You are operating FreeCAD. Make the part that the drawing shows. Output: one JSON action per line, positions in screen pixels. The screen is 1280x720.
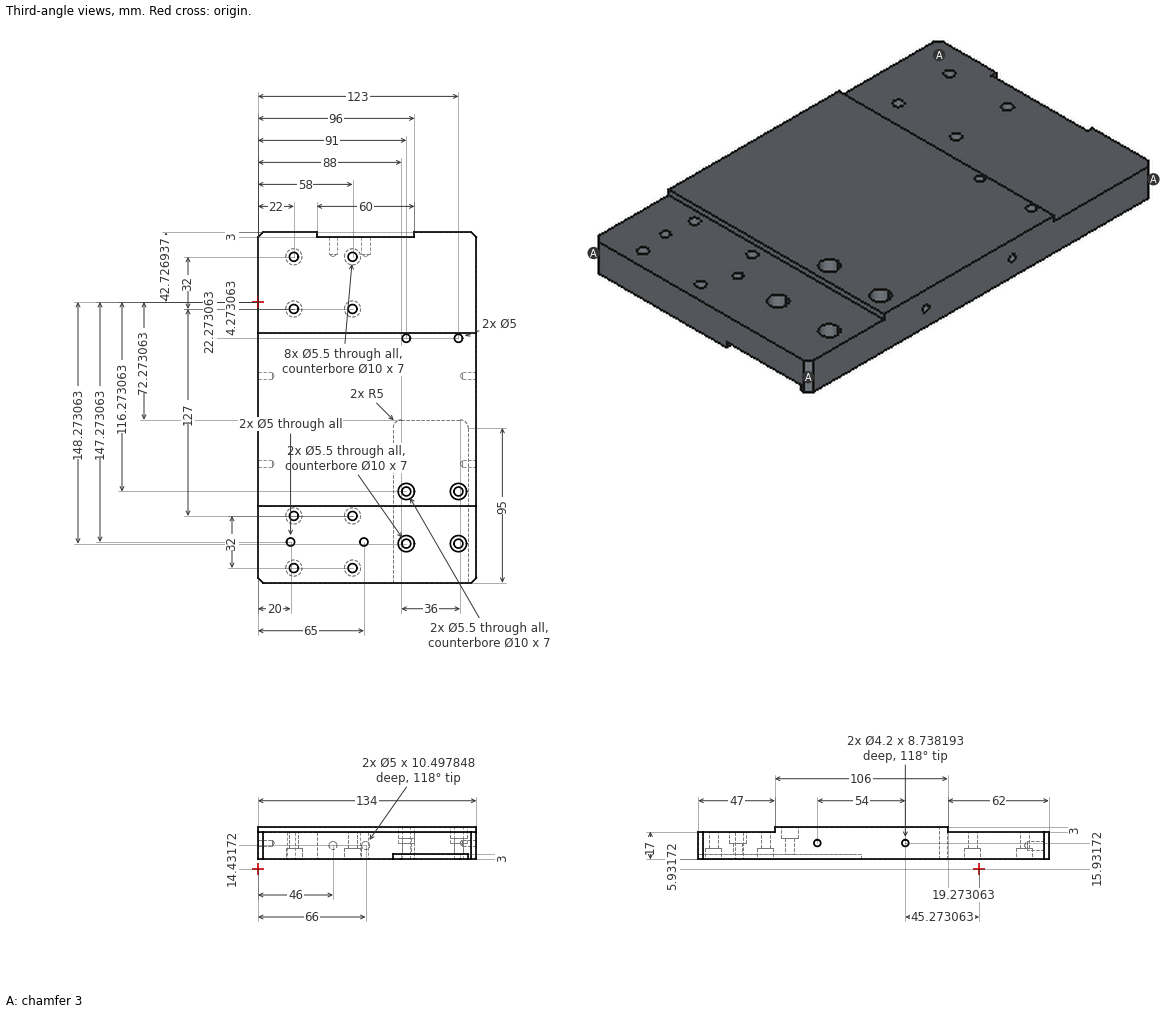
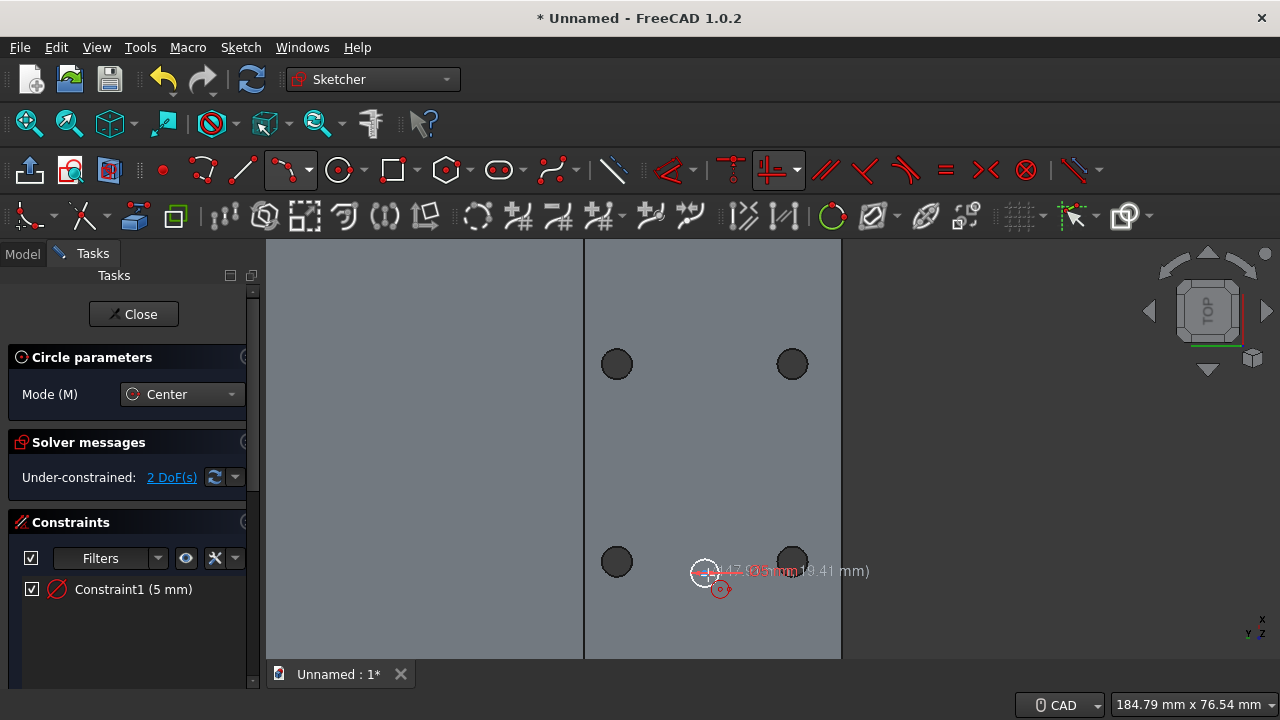
{"action": "scroll", "coordinate": [705, 326], "scroll_direction": "up", "scroll_amount": 3}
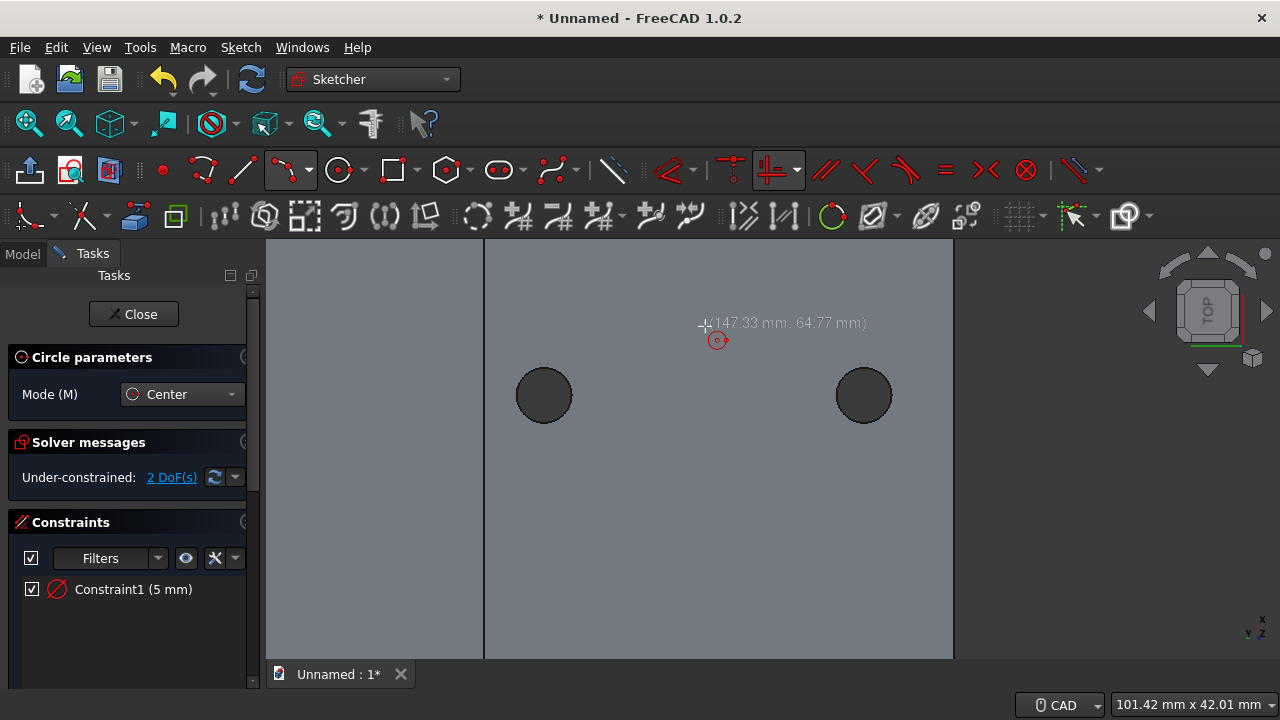
{"action": "left_click", "coordinate": [704, 325]}
{"action": "mouse_move", "coordinate": [722, 308]}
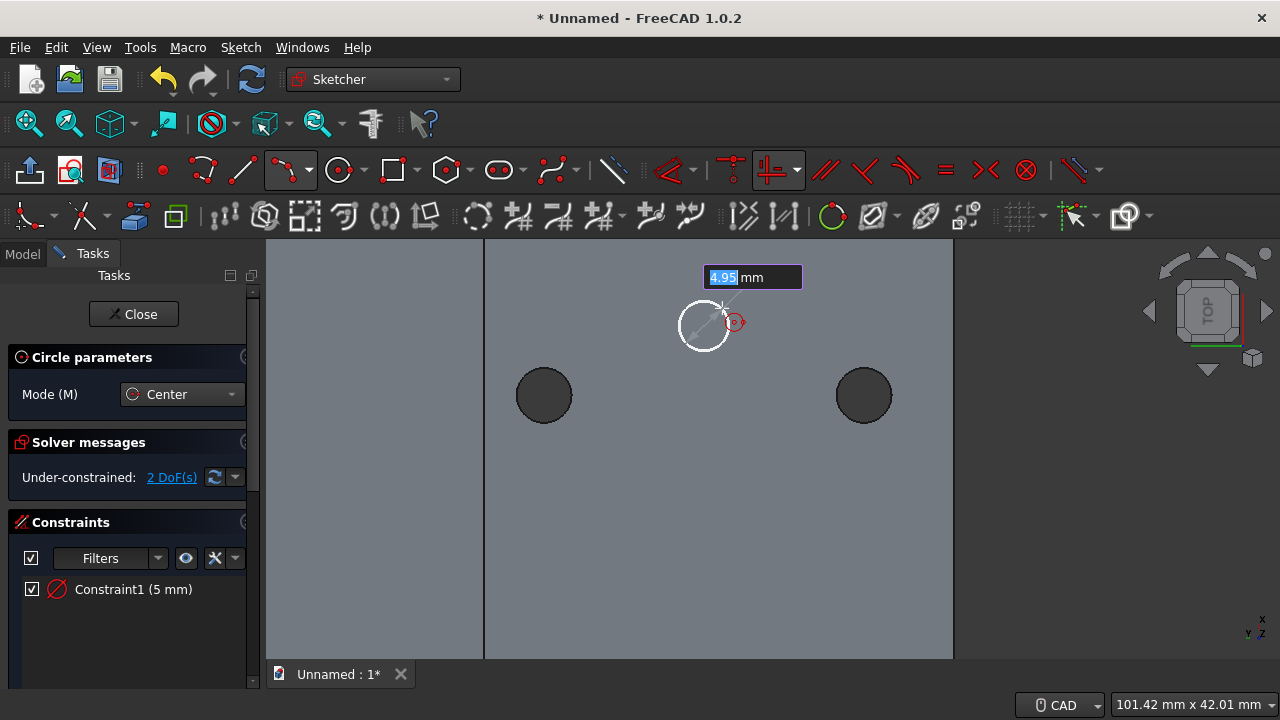
{"action": "type", "text": "5"}
{"action": "key", "text": "Return"}
{"action": "key", "text": "Escape"}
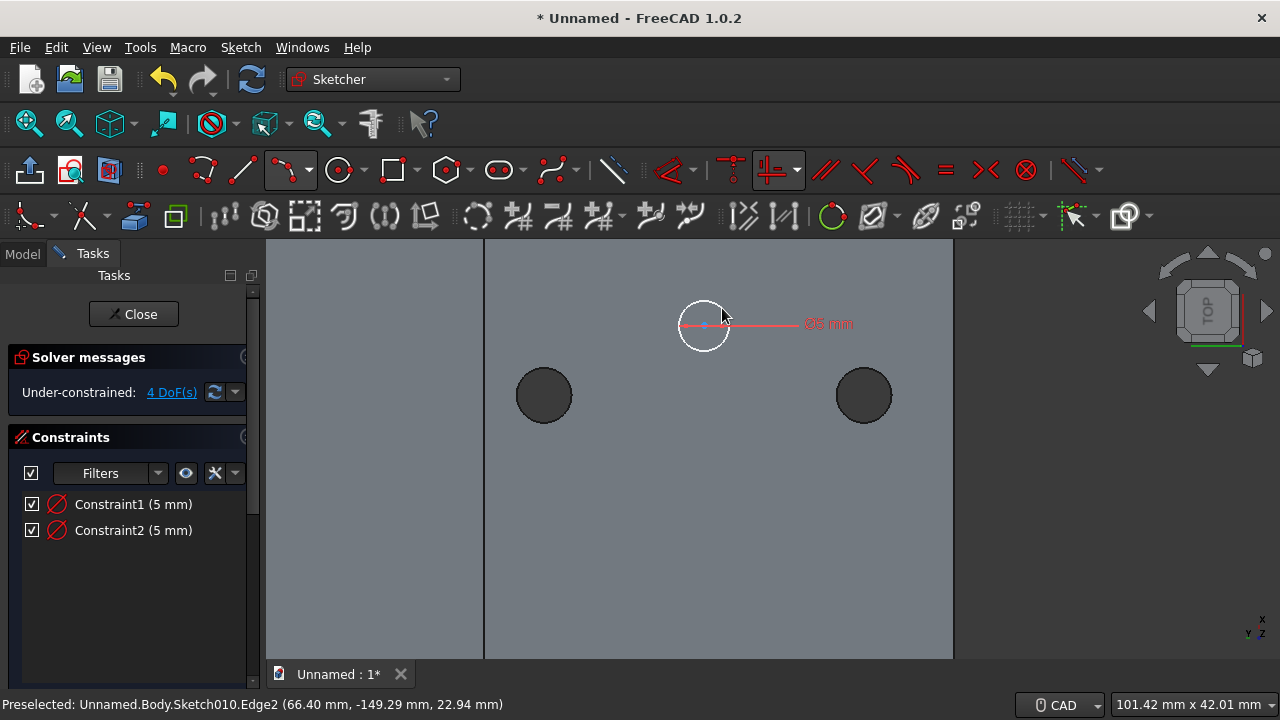
{"action": "scroll", "coordinate": [705, 326], "scroll_direction": "down", "scroll_amount": 3}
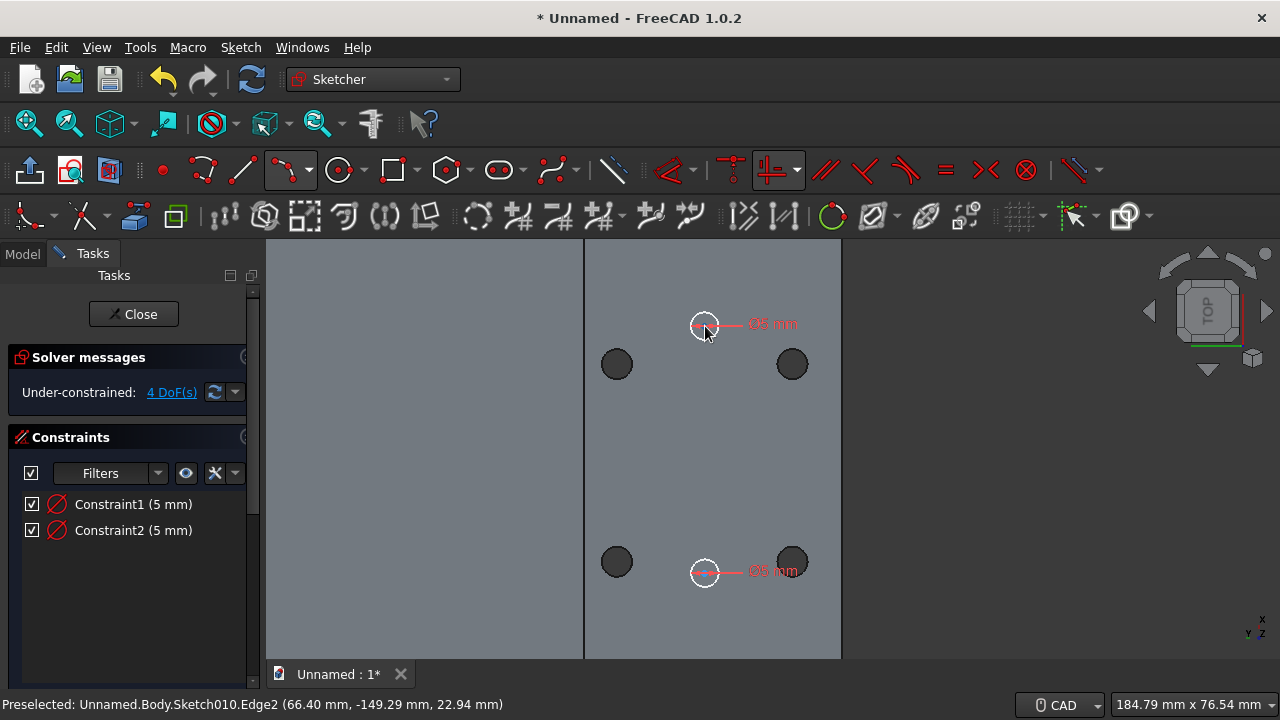
{"action": "left_click", "coordinate": [705, 573]}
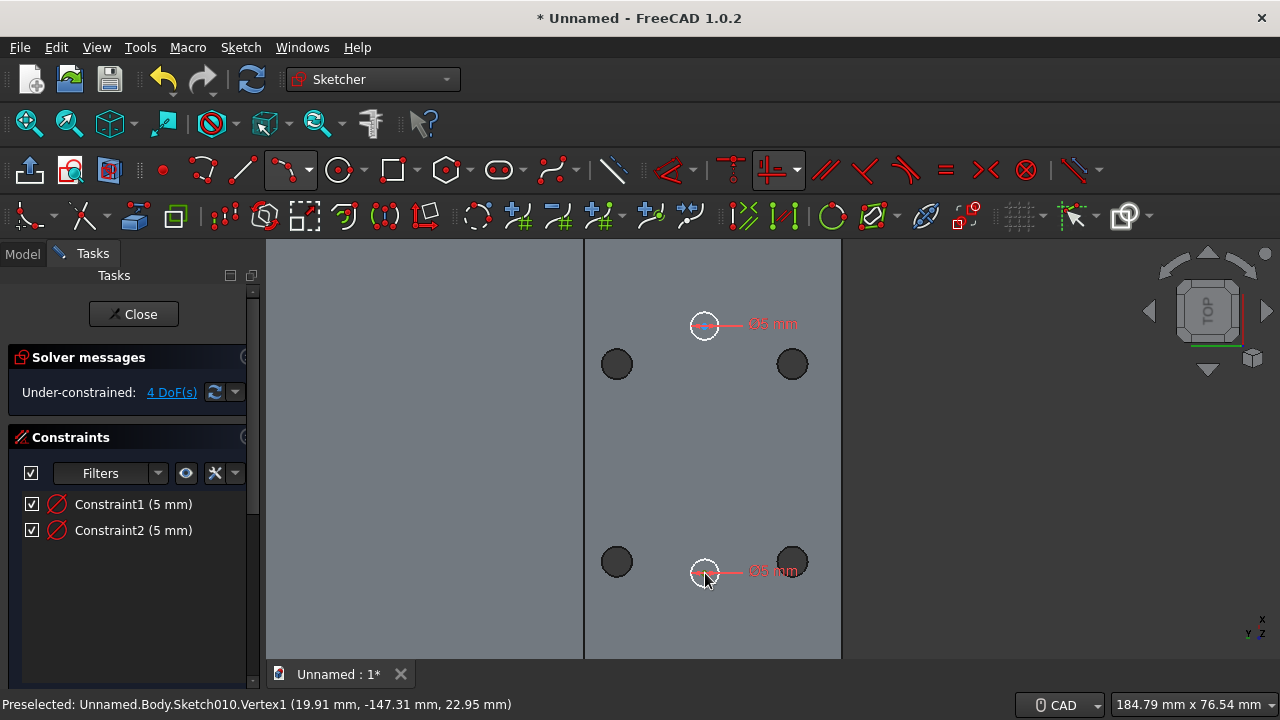
{"action": "left_click", "coordinate": [705, 326]}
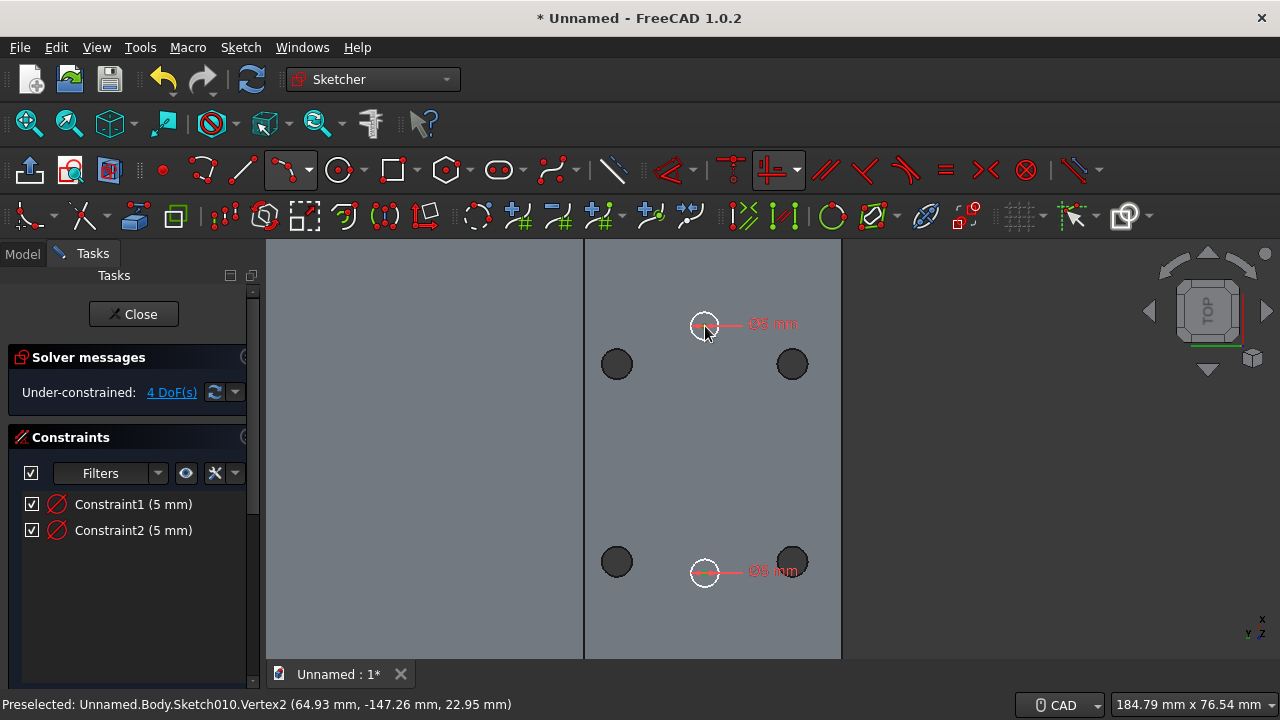
{"action": "key", "text": "v"}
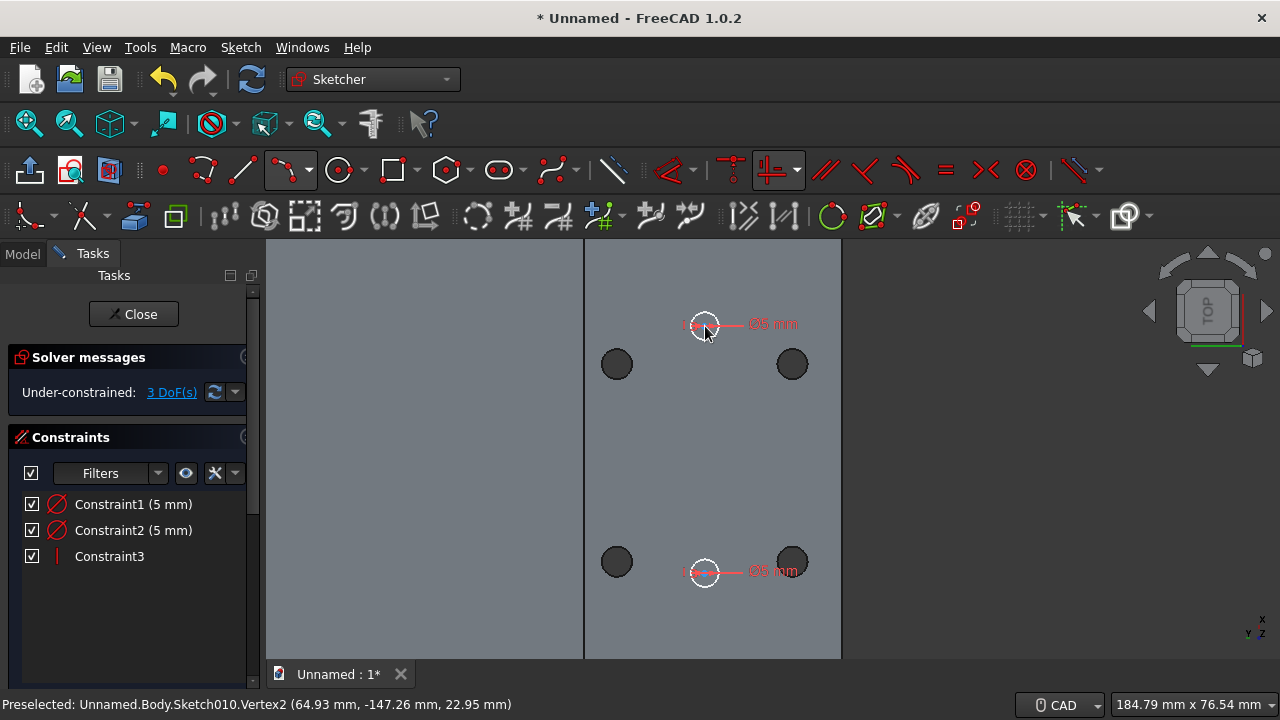
{"action": "left_click", "coordinate": [668, 170]}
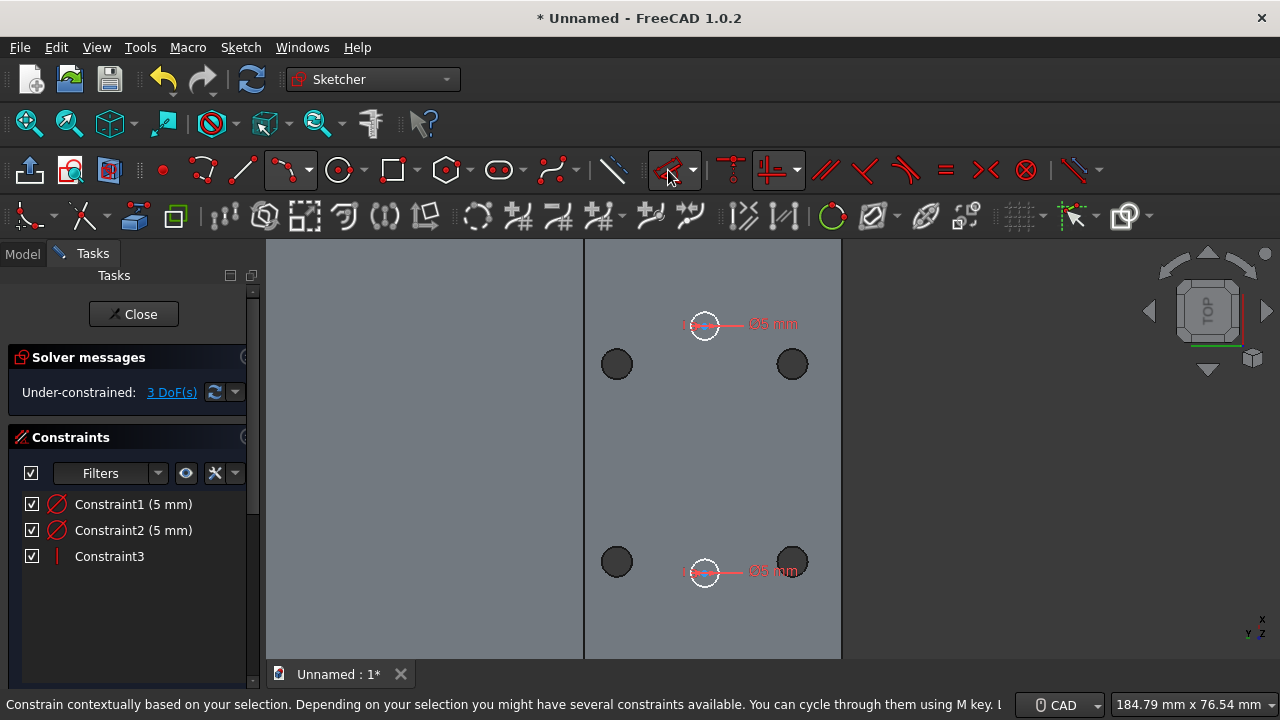
{"action": "left_click", "coordinate": [705, 573]}
{"action": "left_click", "coordinate": [739, 602]}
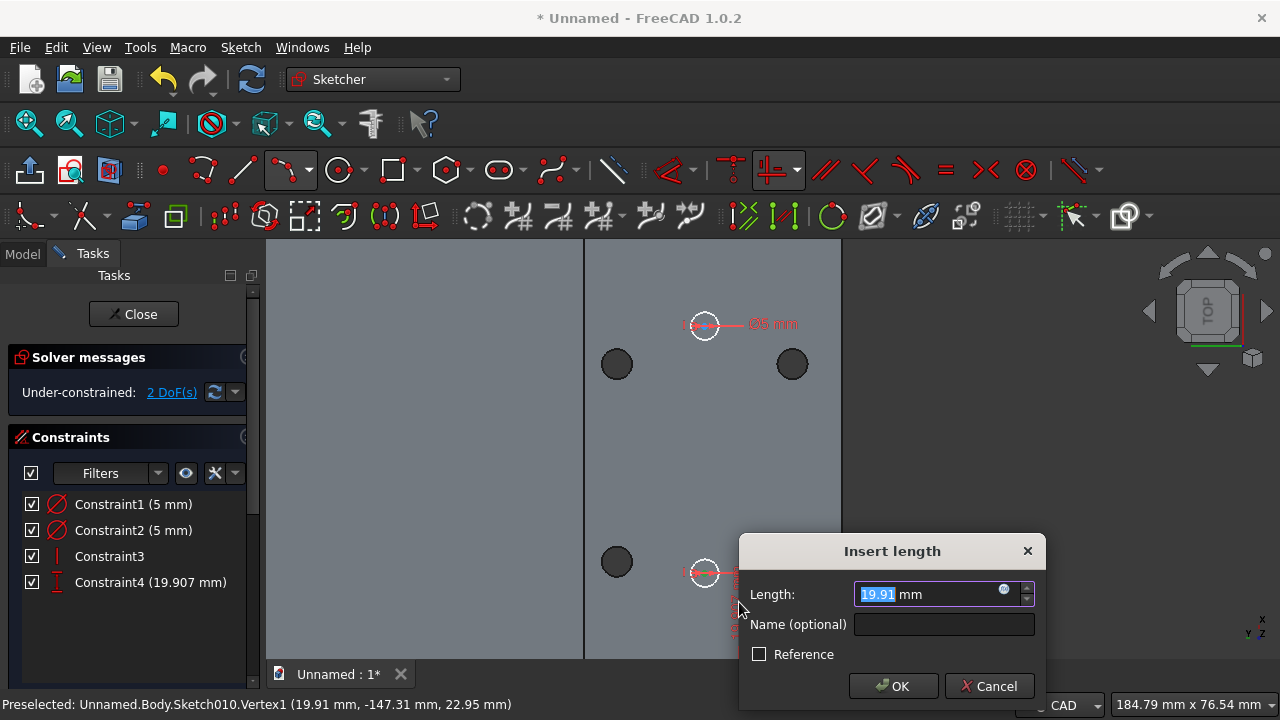
{"action": "type", "text": "20"}
{"action": "key", "text": "Return"}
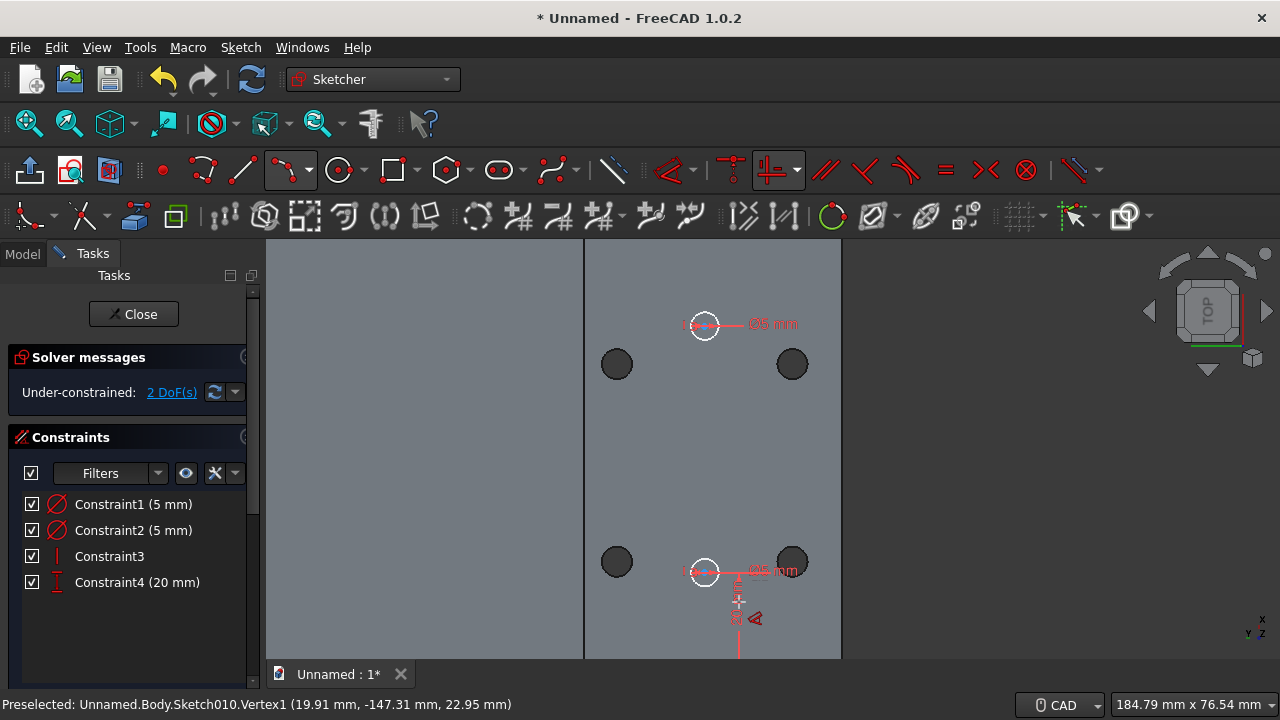
{"action": "left_click", "coordinate": [705, 326]}
{"action": "left_click", "coordinate": [739, 479]}